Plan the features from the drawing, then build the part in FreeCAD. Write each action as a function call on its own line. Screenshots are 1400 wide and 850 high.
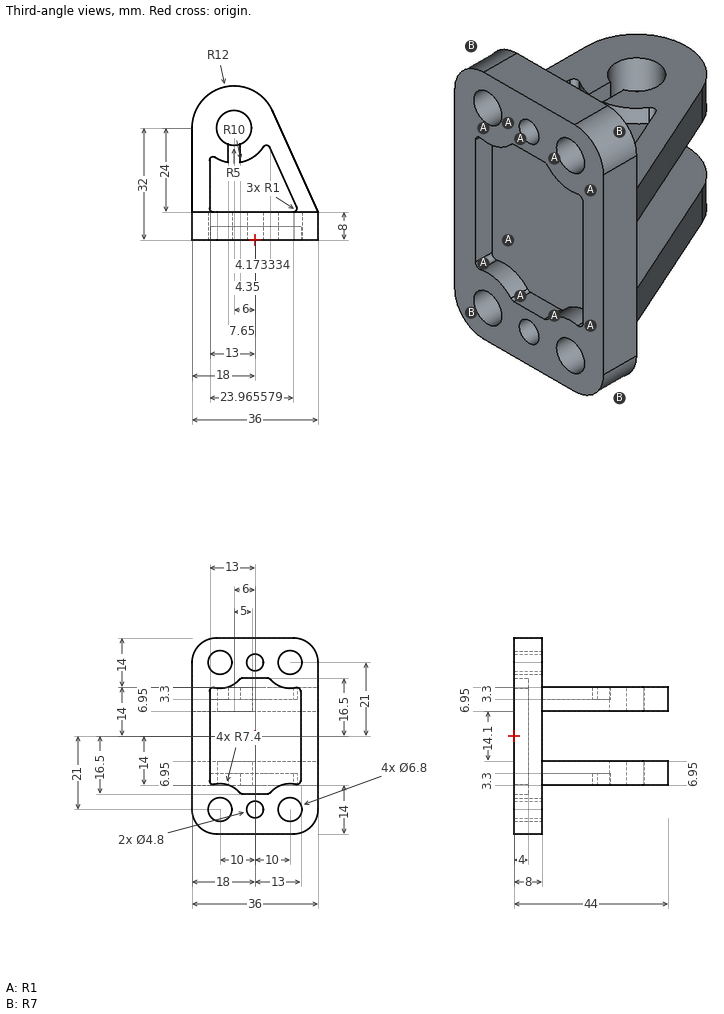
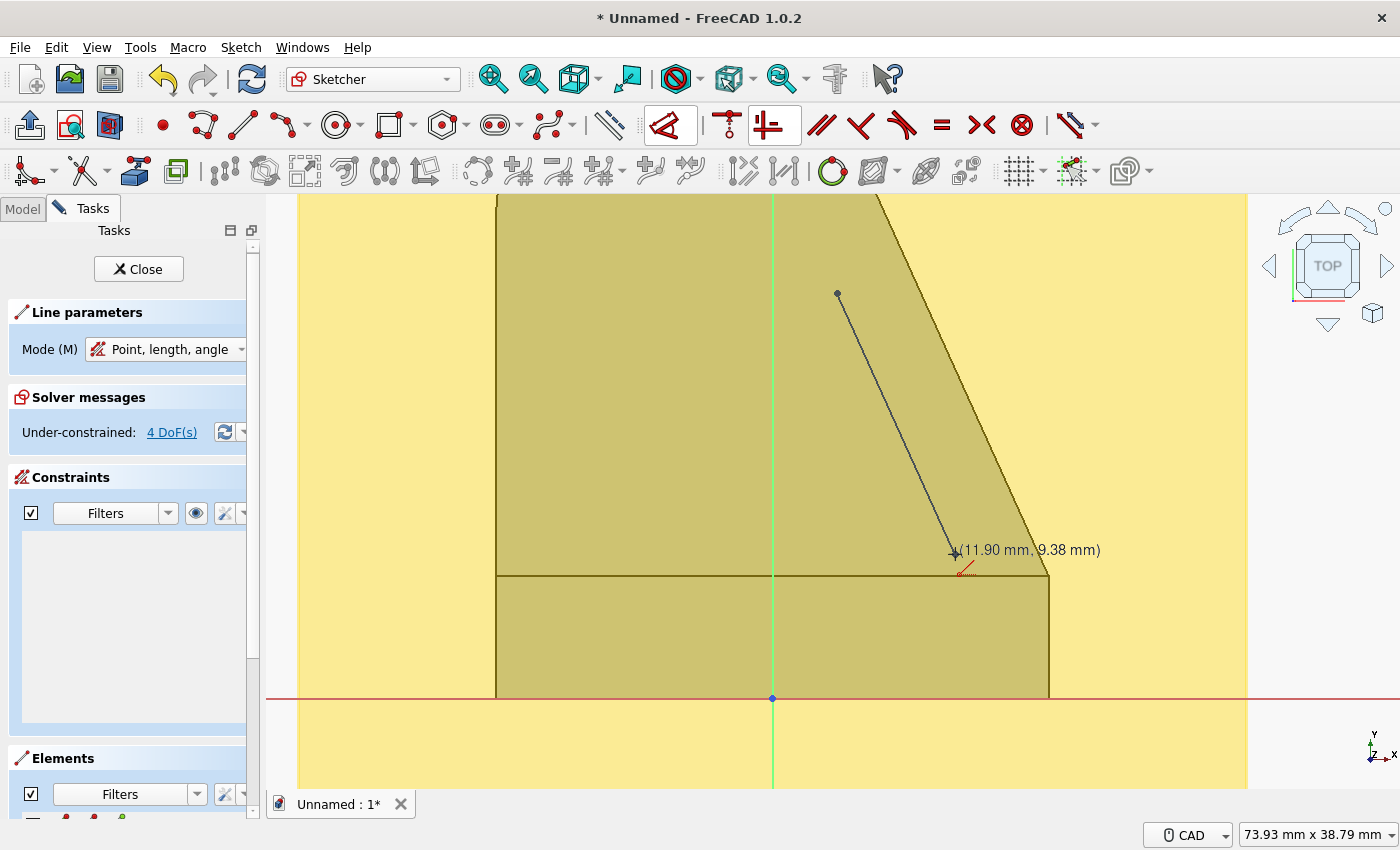
key(g)
key(m)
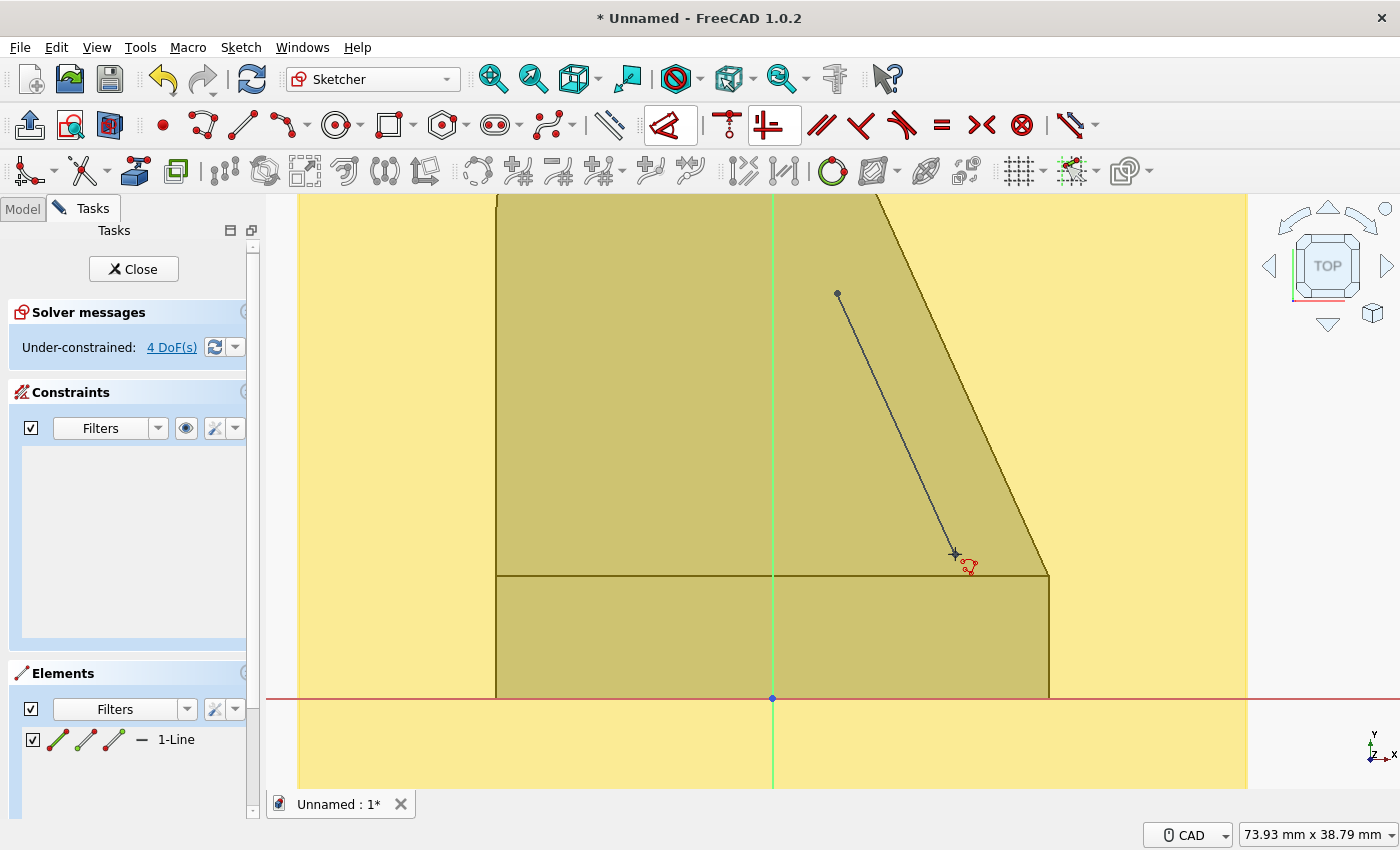
click(941, 576)
click(573, 576)
click(573, 349)
right_click(573, 349)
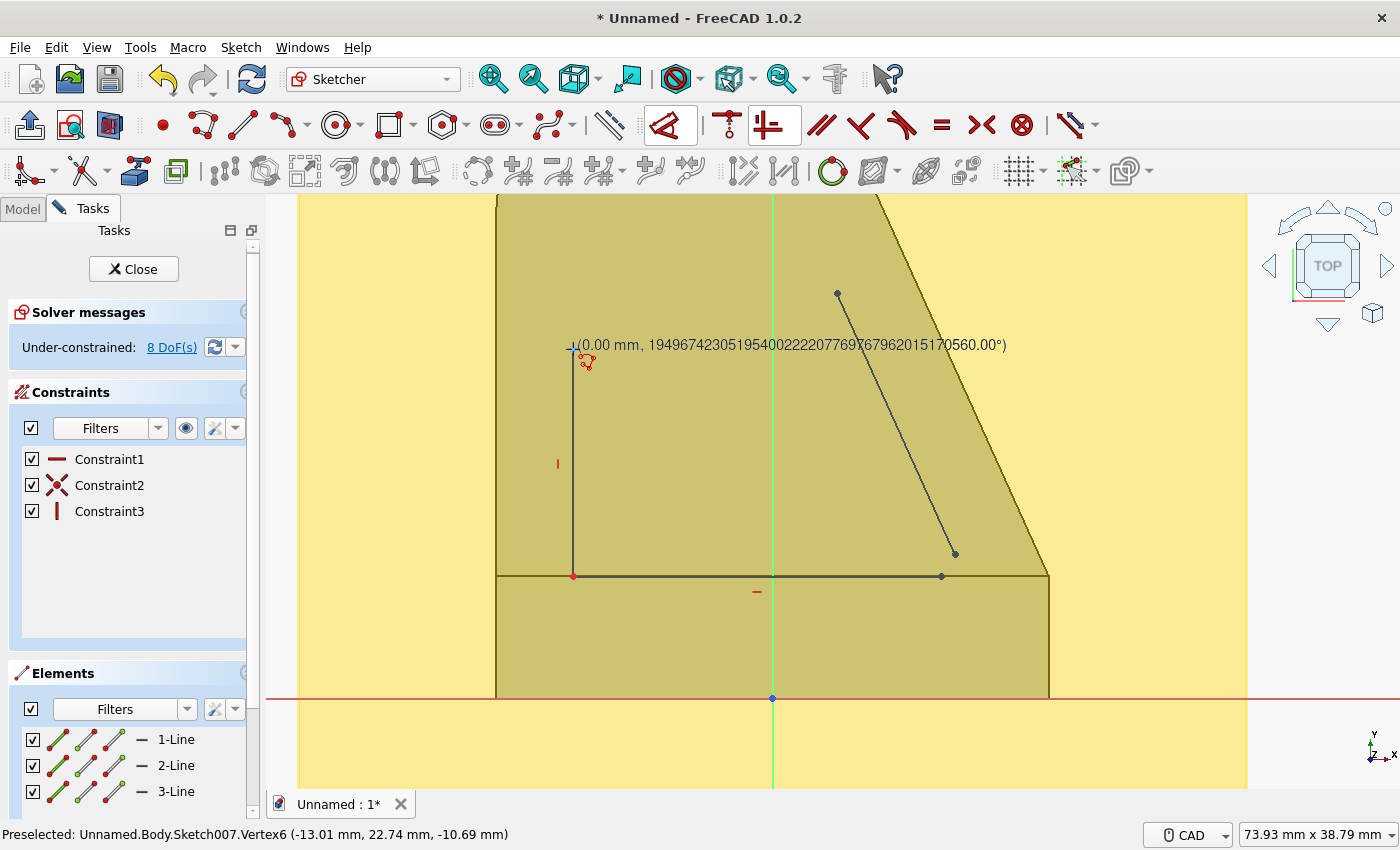
key(g)
key(3)
key(a)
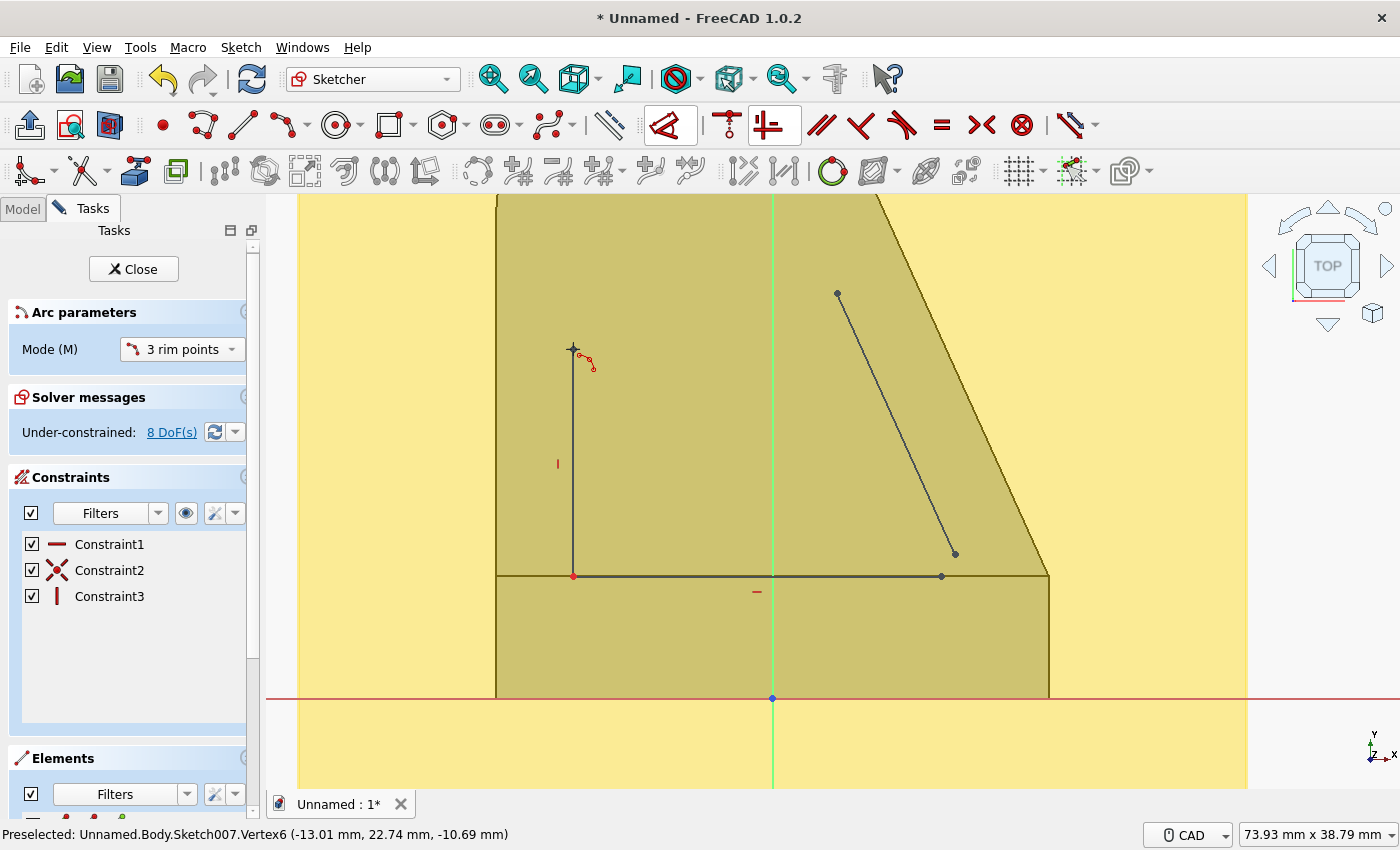
click(955, 555)
click(941, 577)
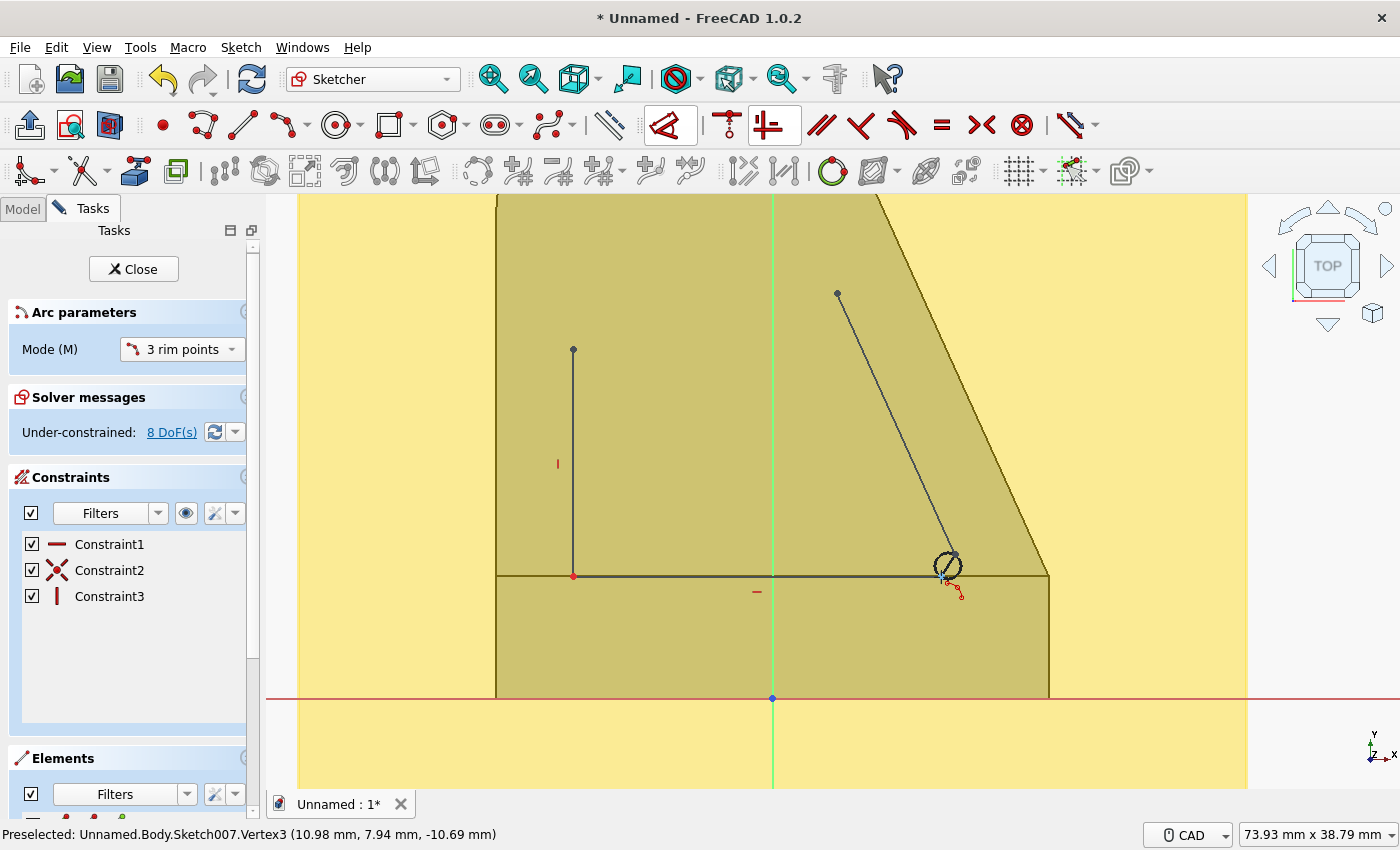
scroll(954, 569, up, 5)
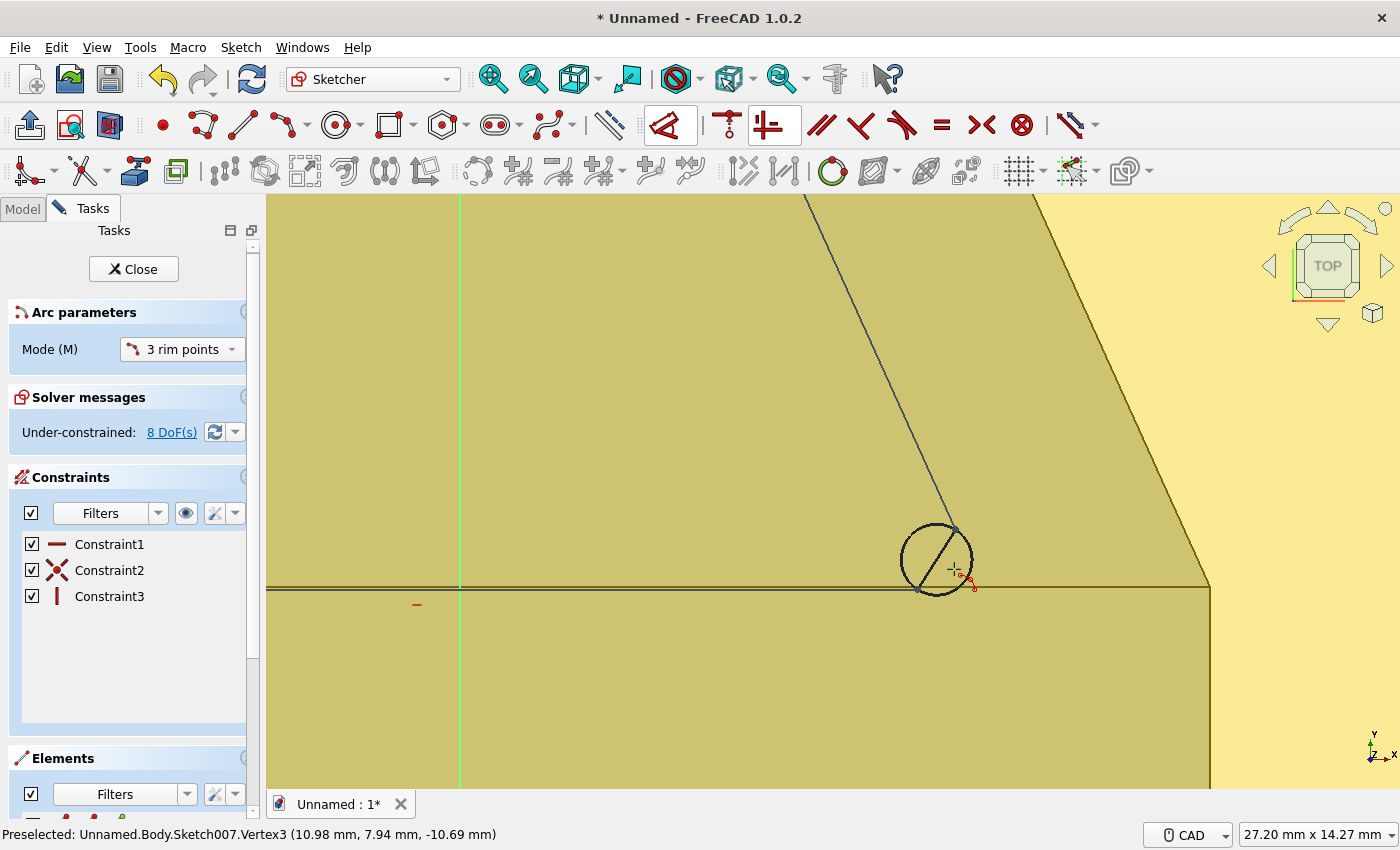
click(952, 568)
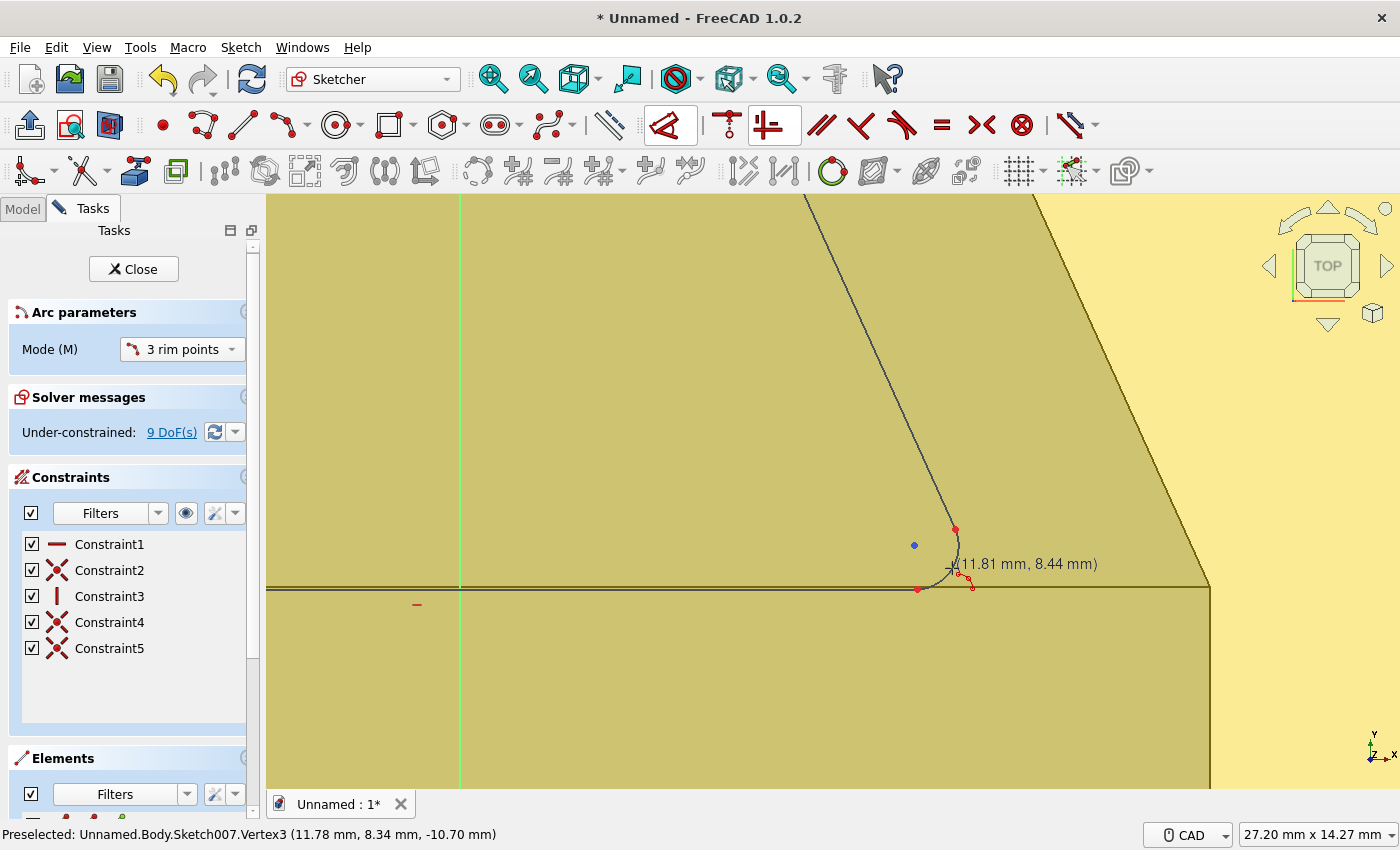
scroll(956, 570, down, 5)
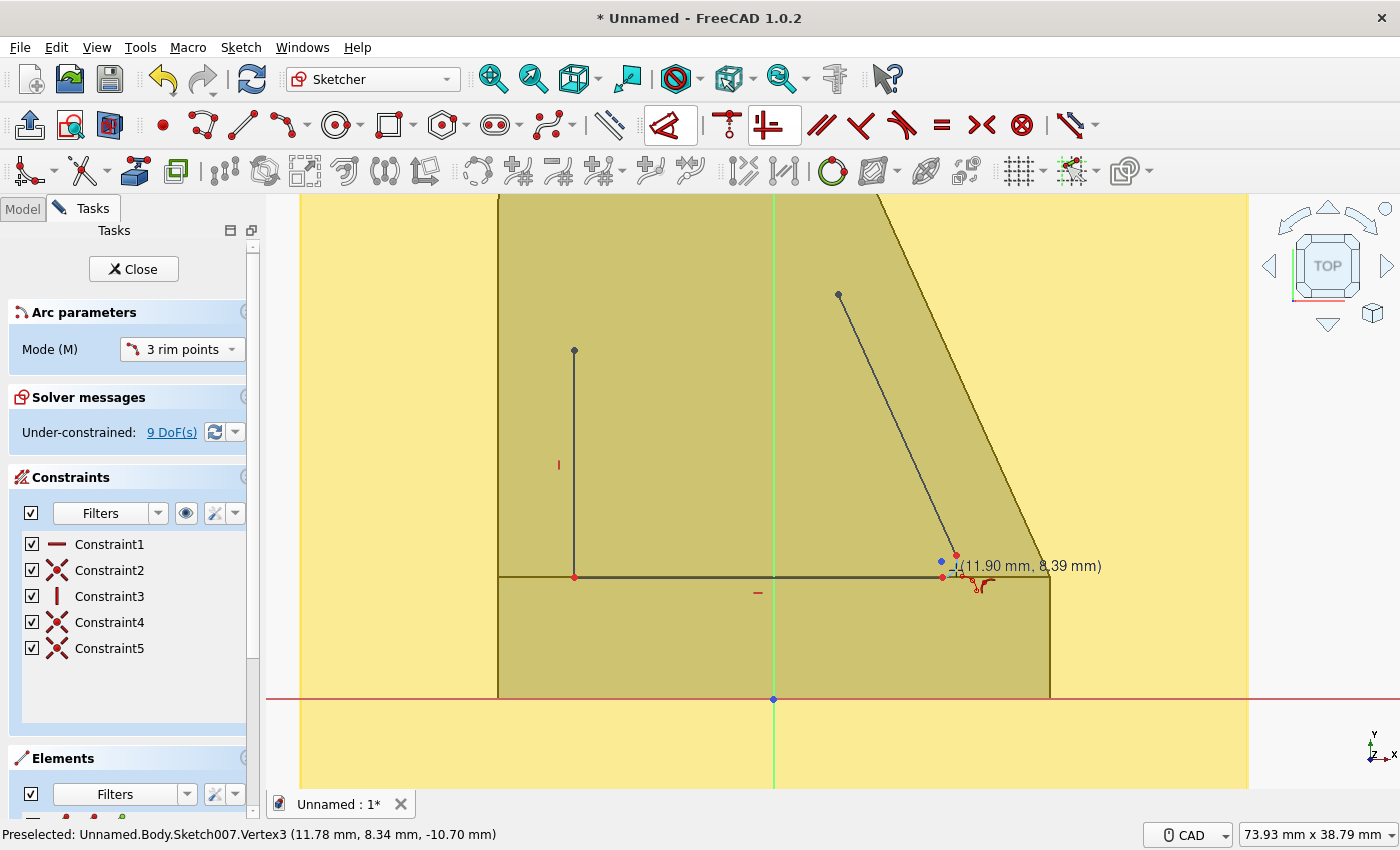
click(574, 351)
click(598, 337)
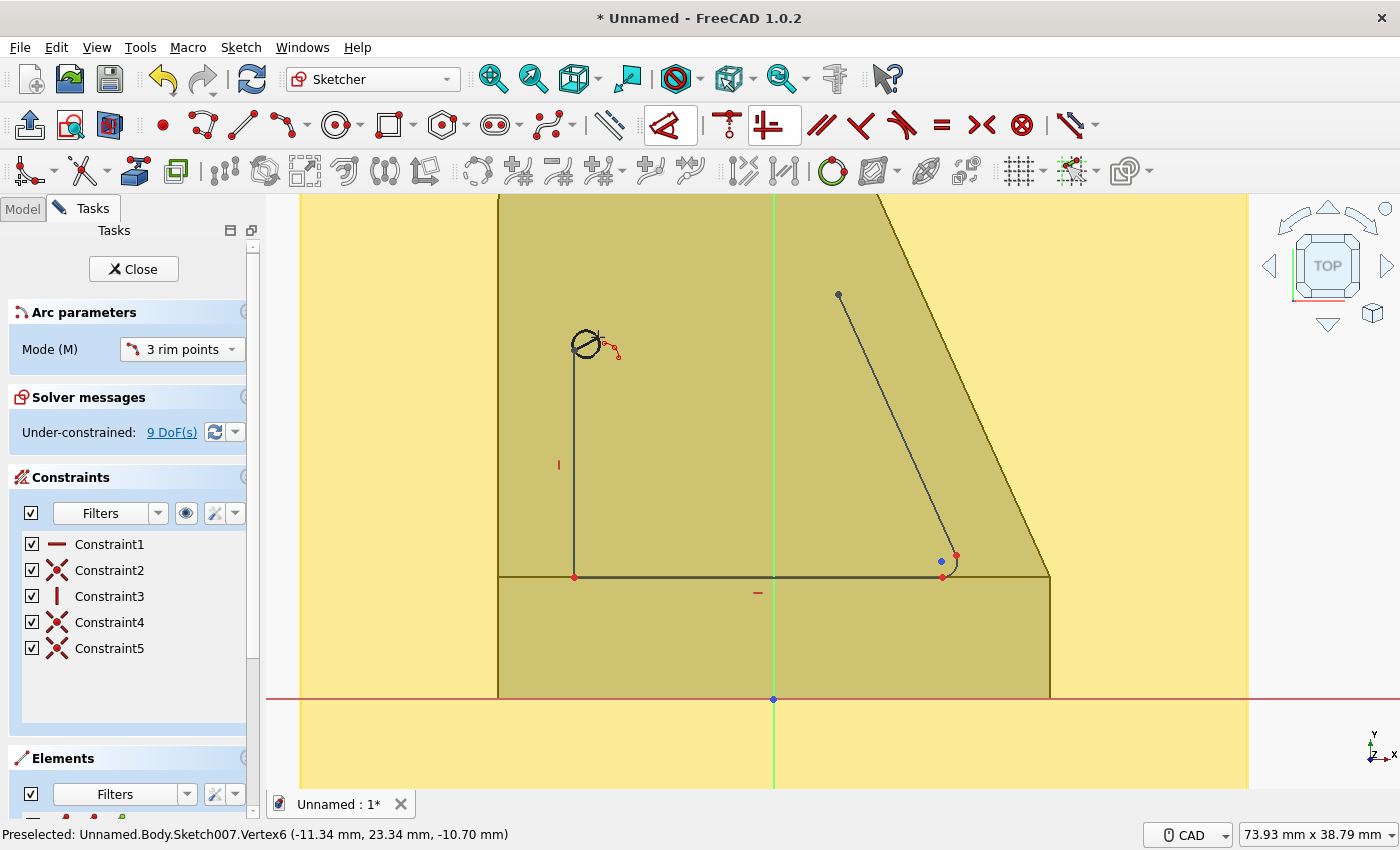
scroll(582, 337, up, 4)